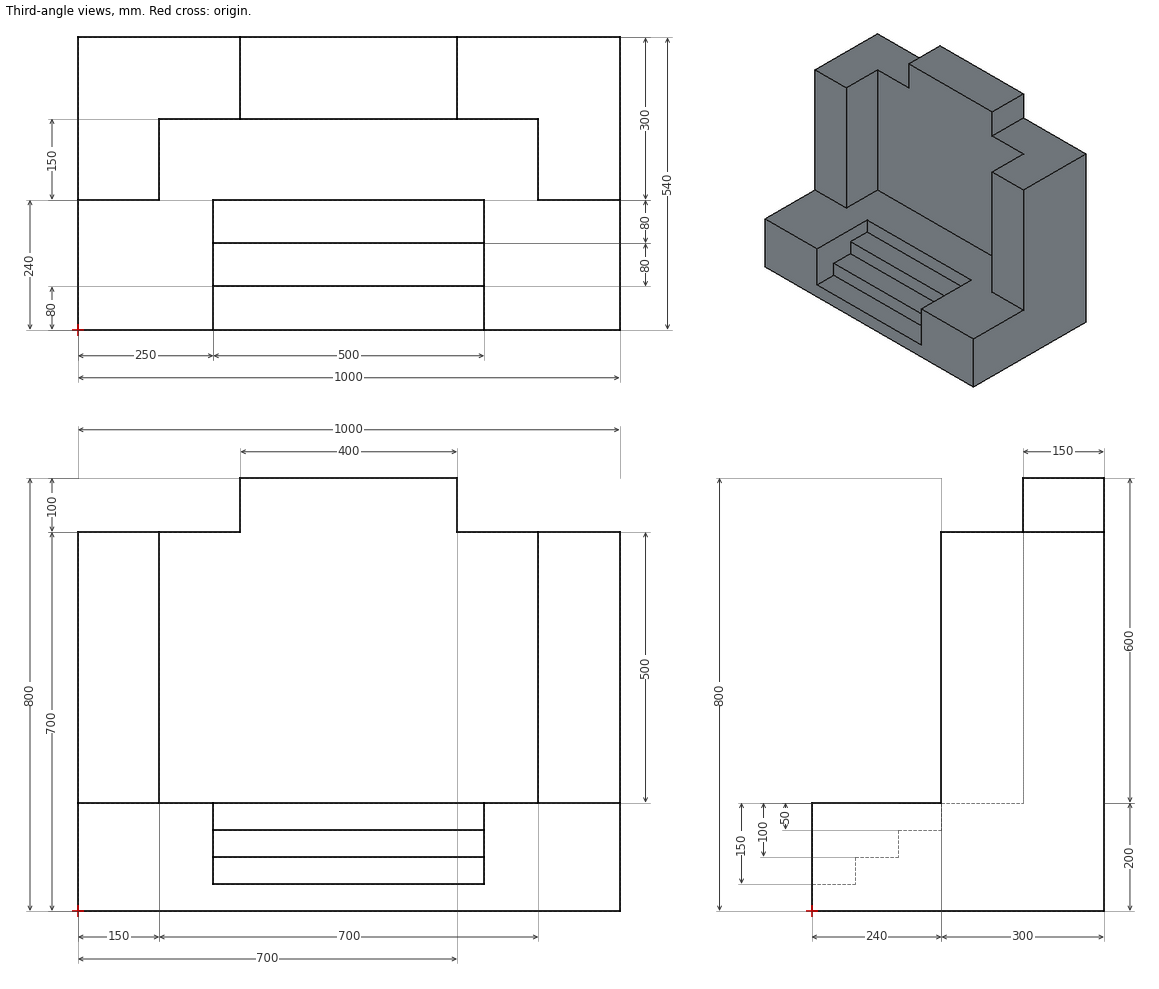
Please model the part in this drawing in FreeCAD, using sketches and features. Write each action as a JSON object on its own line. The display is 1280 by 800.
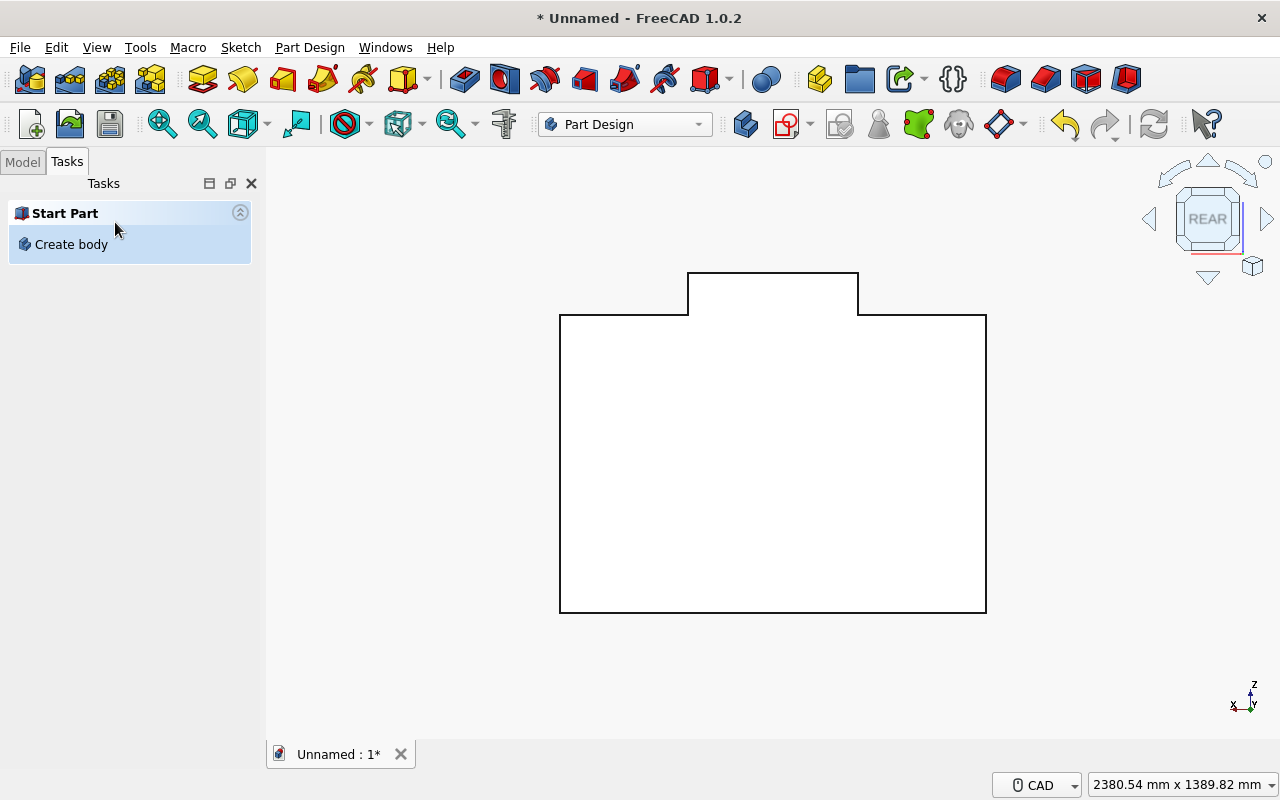
{"action": "key", "text": "0"}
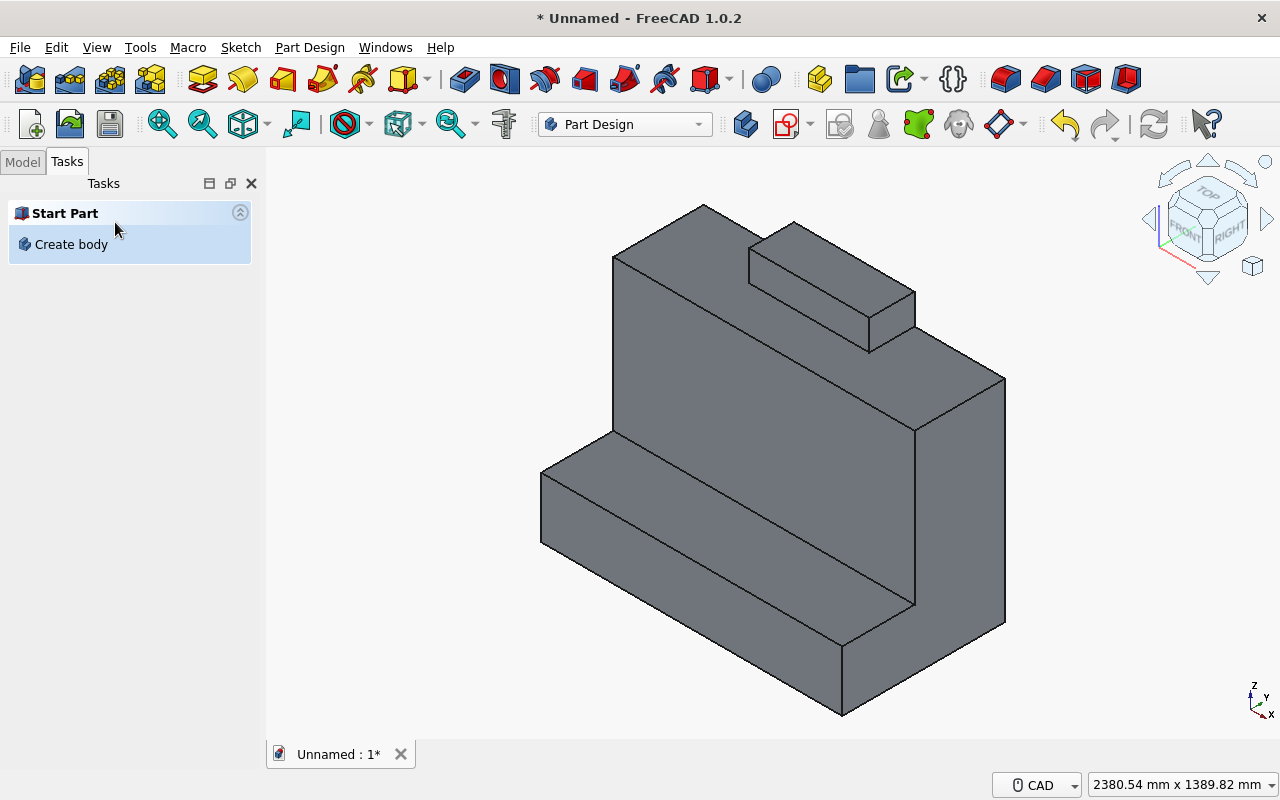
{"action": "left_click", "coordinate": [807, 455]}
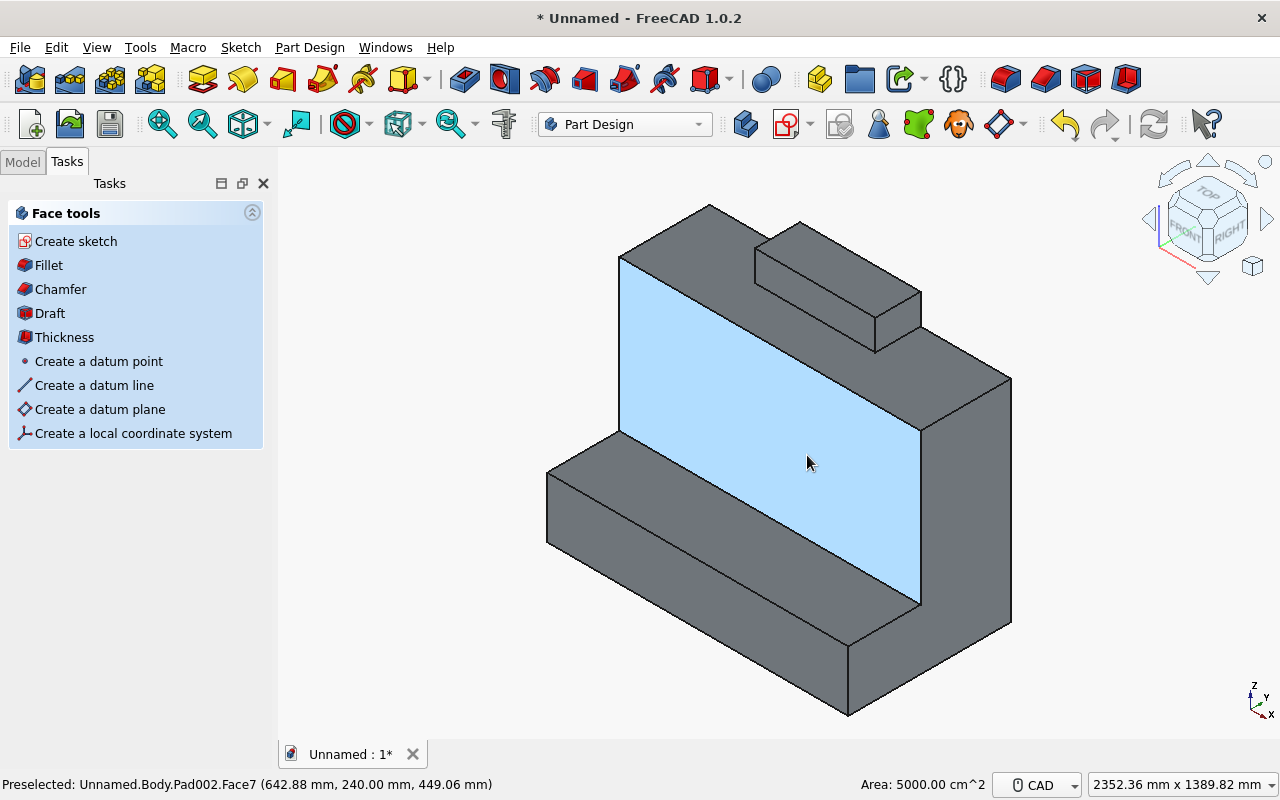
{"action": "left_click", "coordinate": [786, 124]}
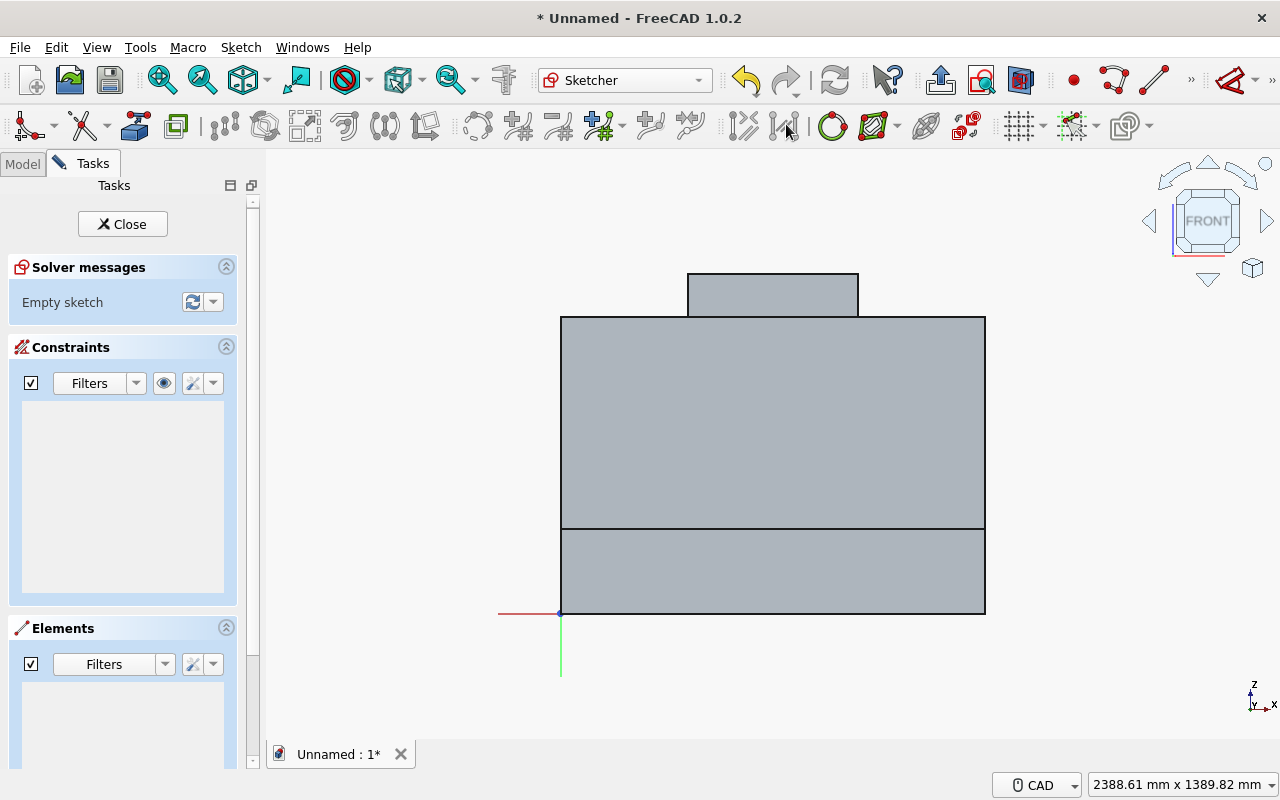
{"action": "left_click", "coordinate": [1022, 80]}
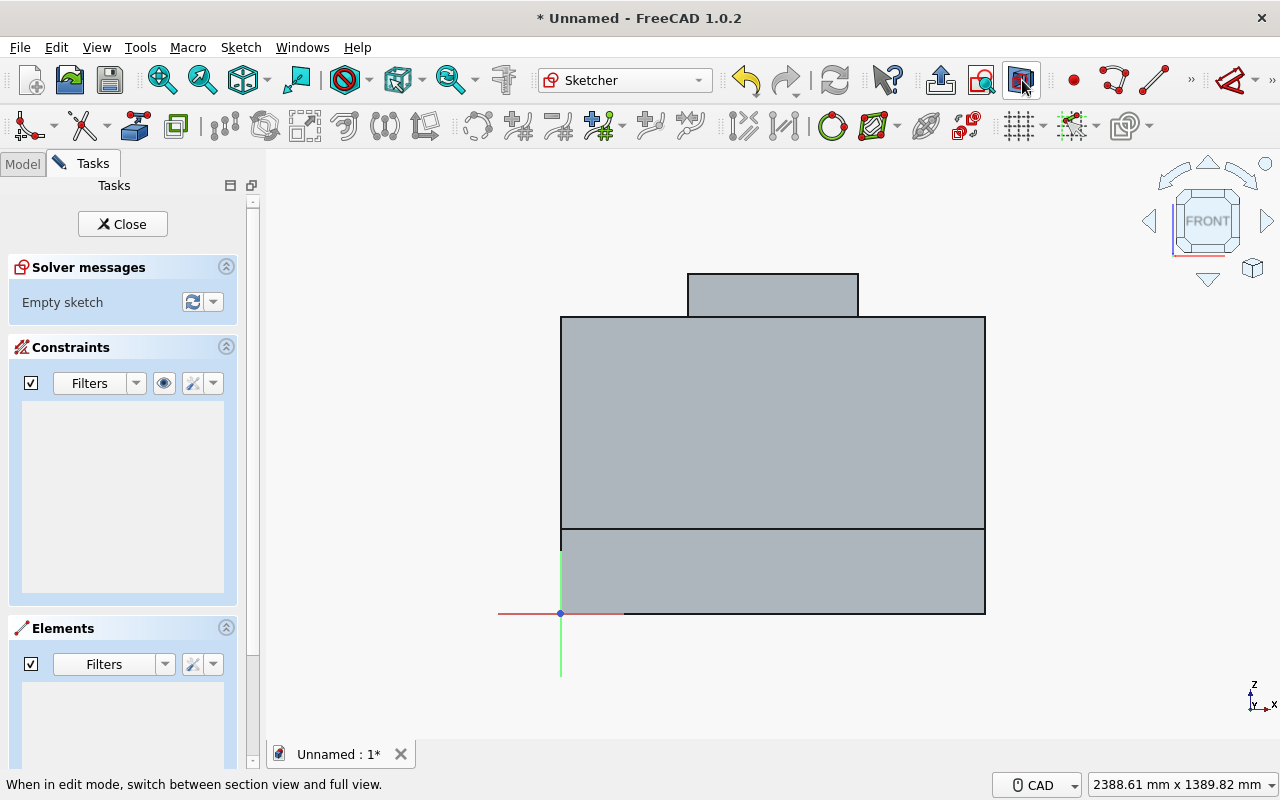
{"action": "key", "text": "g r"}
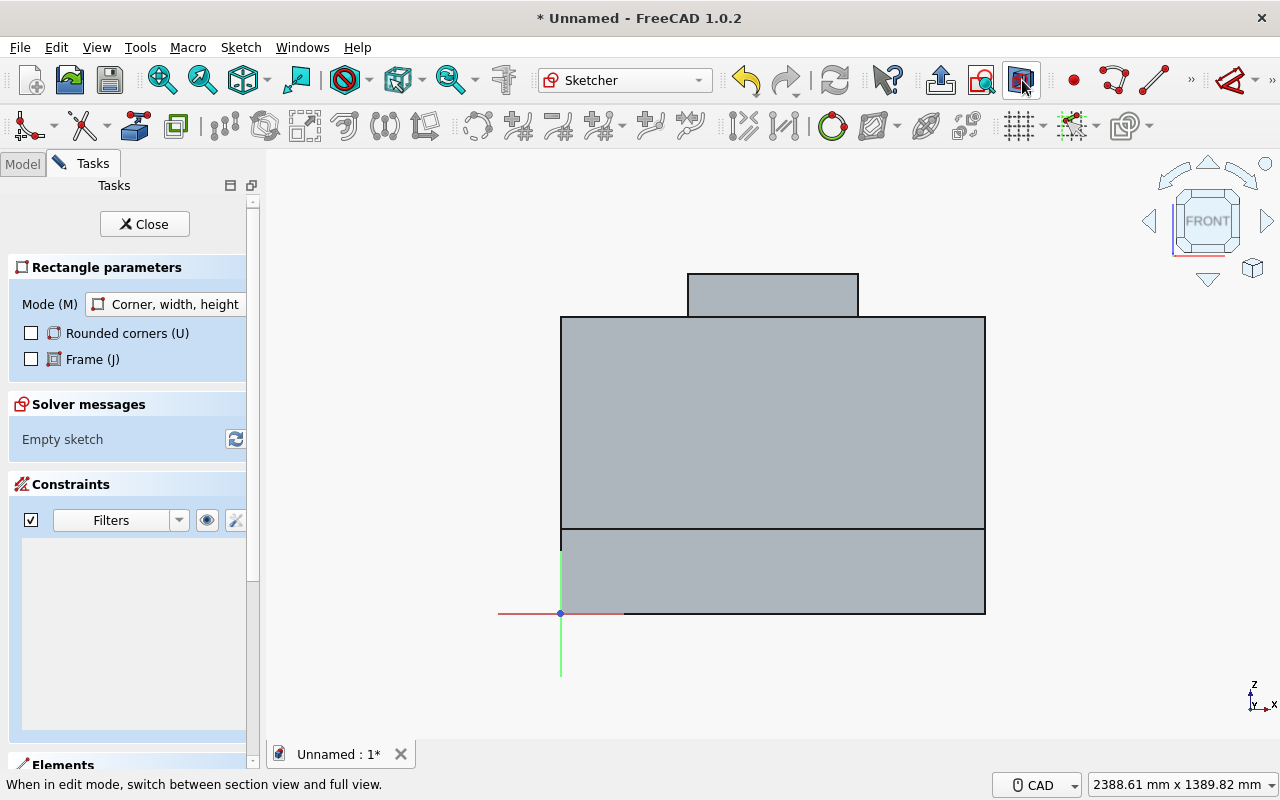
{"action": "left_click", "coordinate": [624, 317]}
{"action": "mouse_move", "coordinate": [922, 529]}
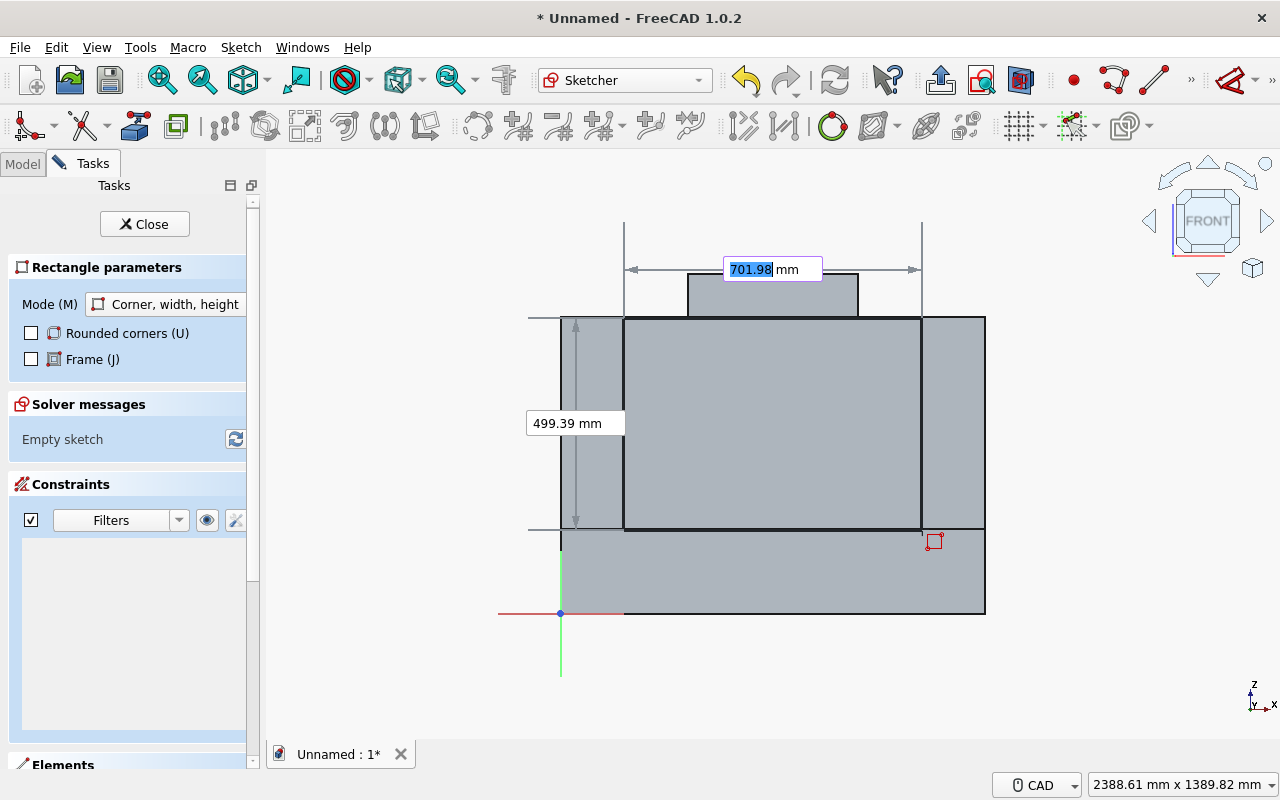
{"action": "type", "text": "700"}
{"action": "key", "text": "Tab"}
{"action": "type", "text": "500"}
{"action": "key", "text": "Return"}
{"action": "key", "text": "Escape"}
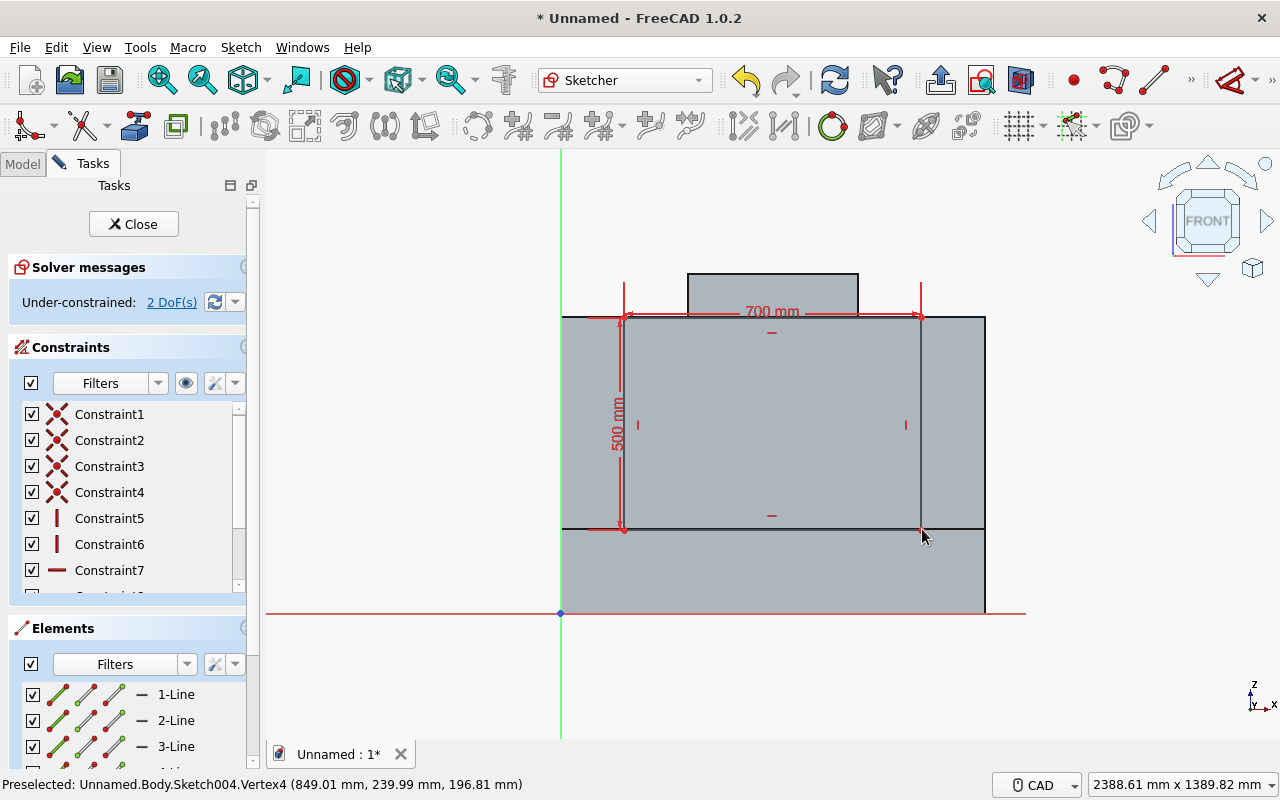
{"action": "left_click", "coordinate": [1230, 80]}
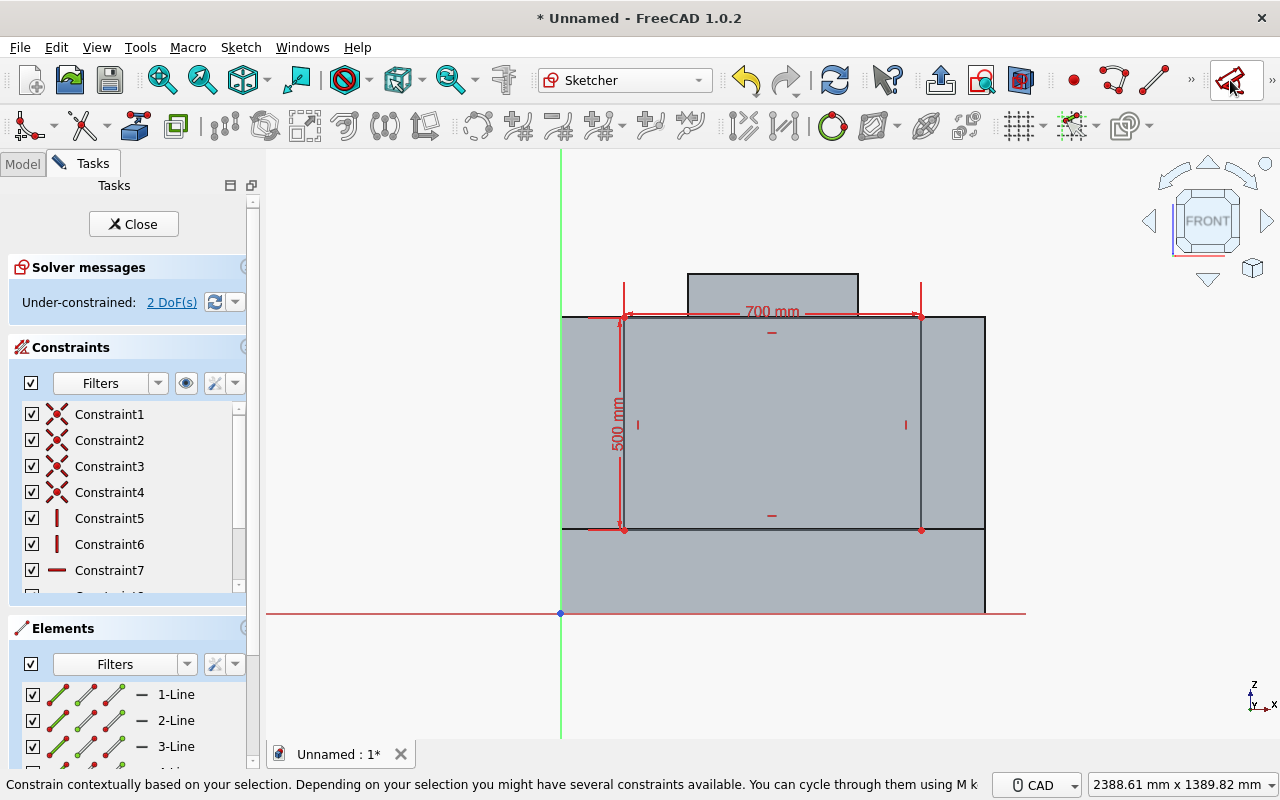
{"action": "left_click", "coordinate": [624, 318]}
{"action": "left_click", "coordinate": [592, 648]}